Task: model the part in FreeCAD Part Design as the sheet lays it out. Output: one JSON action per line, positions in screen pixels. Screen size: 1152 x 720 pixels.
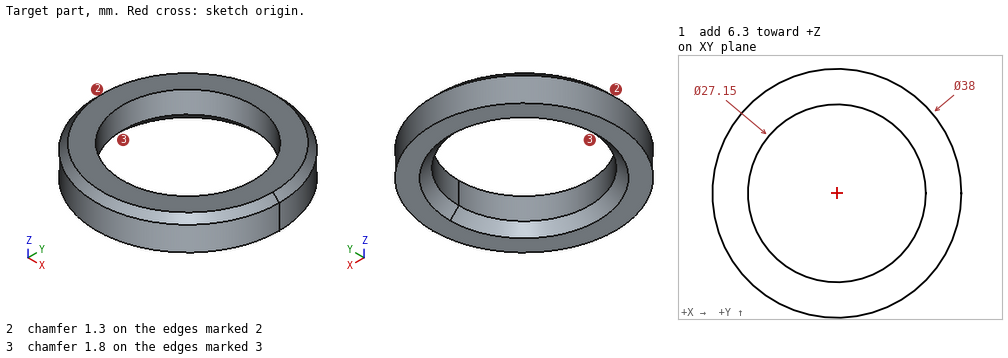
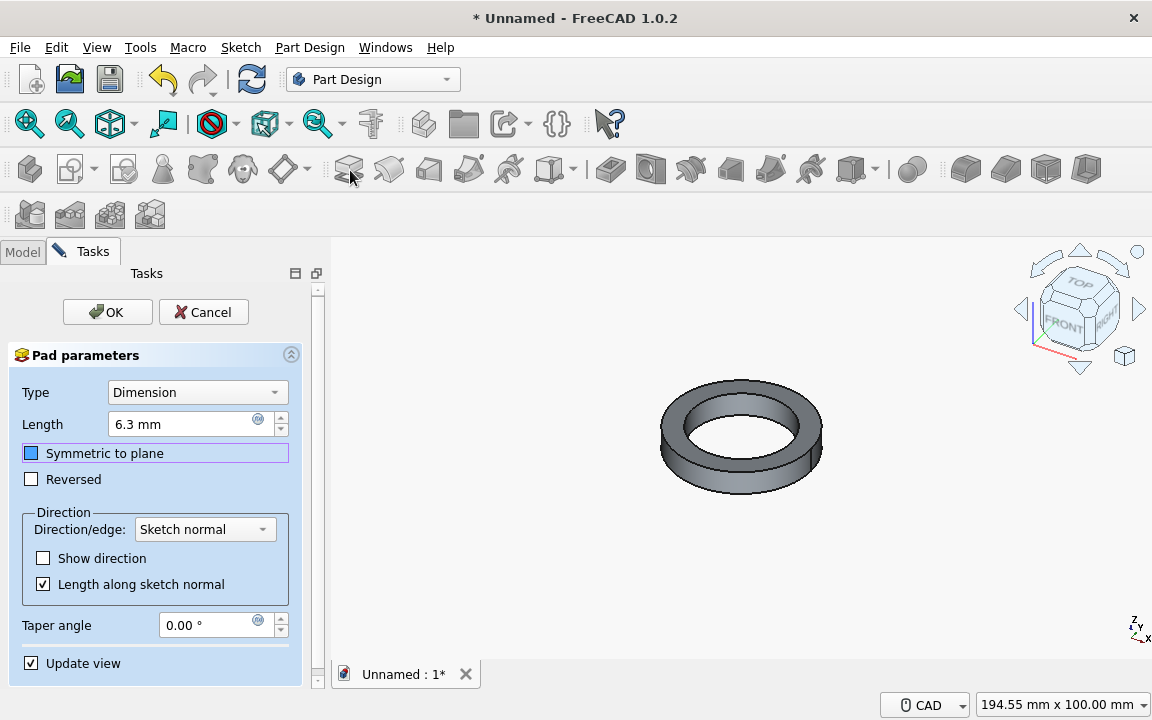
{"action": "left_click", "coordinate": [108, 312]}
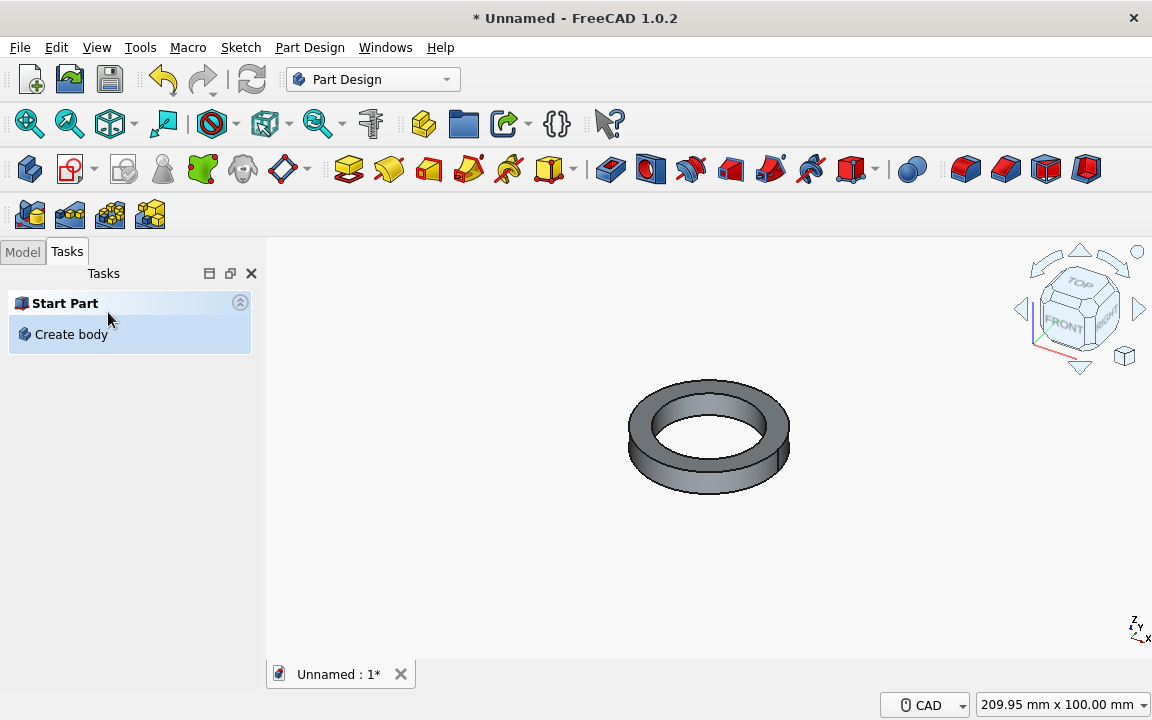
{"action": "key", "text": "v f"}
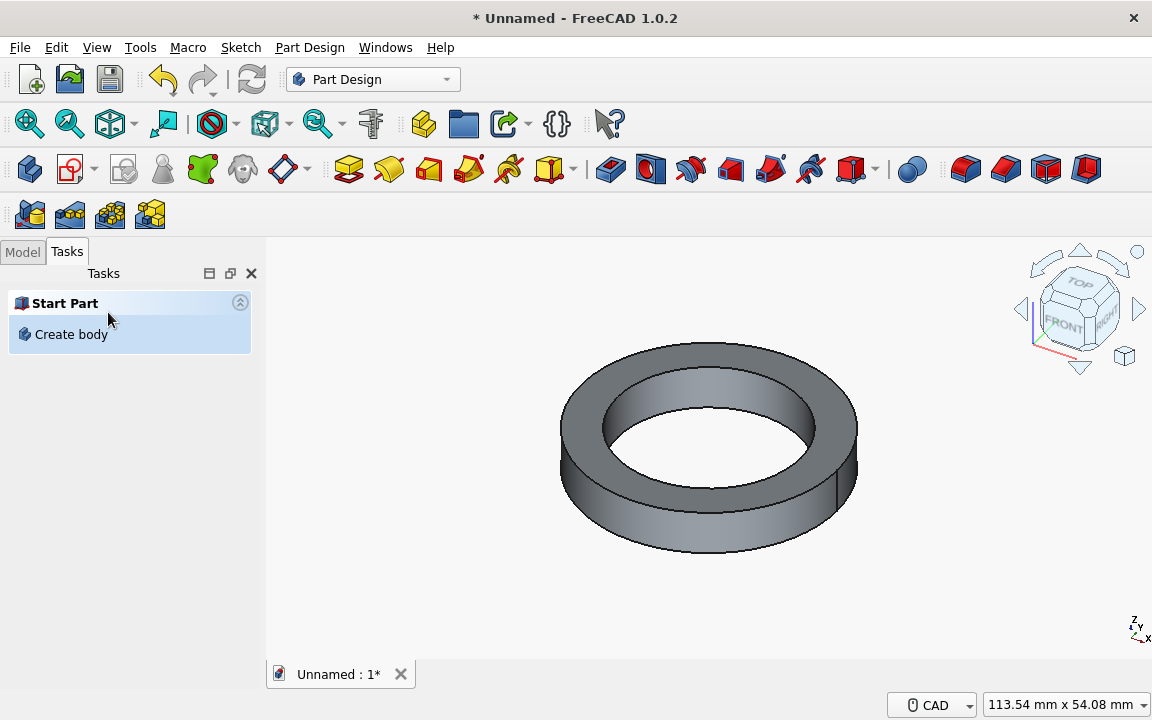
{"action": "left_click", "coordinate": [561, 436]}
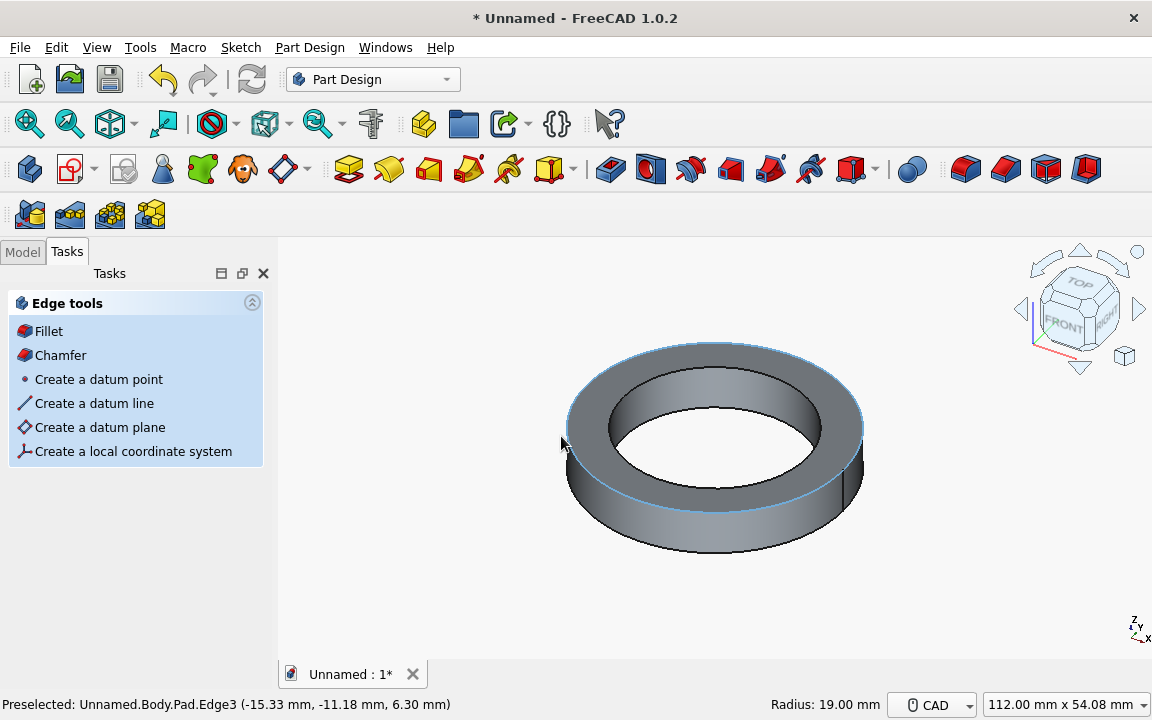
{"action": "left_click", "coordinate": [1006, 170]}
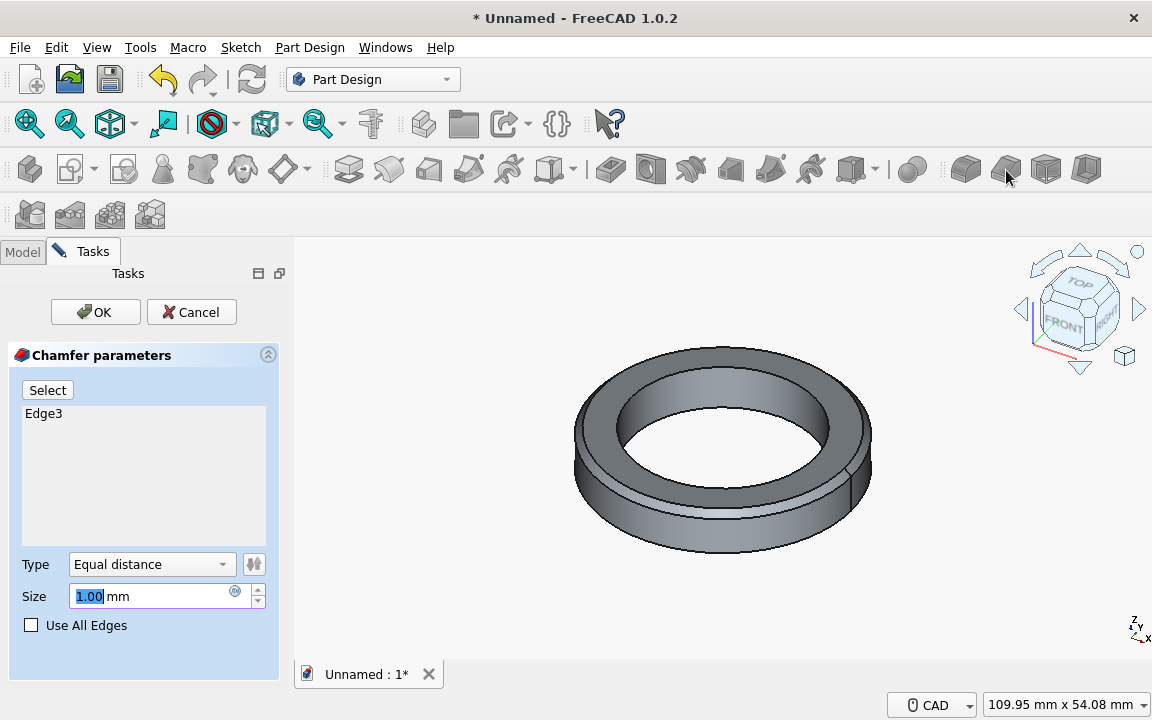
{"action": "type", "text": "1.3"}
{"action": "key", "text": "Tab"}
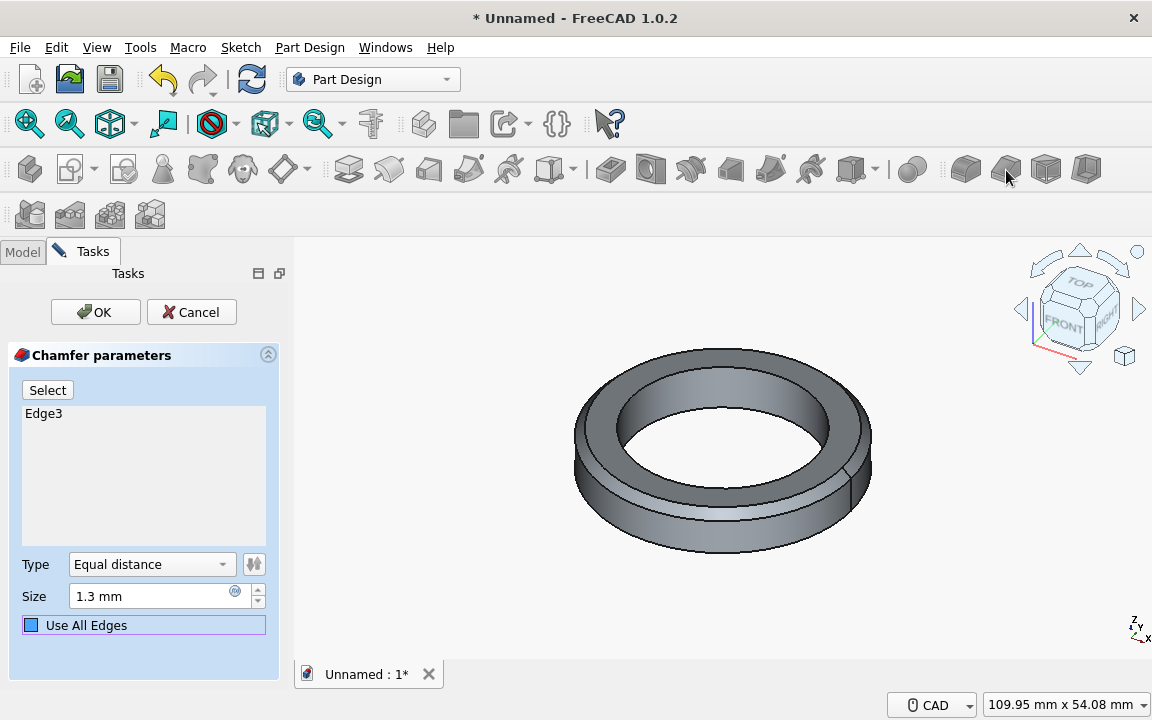
{"action": "left_click", "coordinate": [96, 312]}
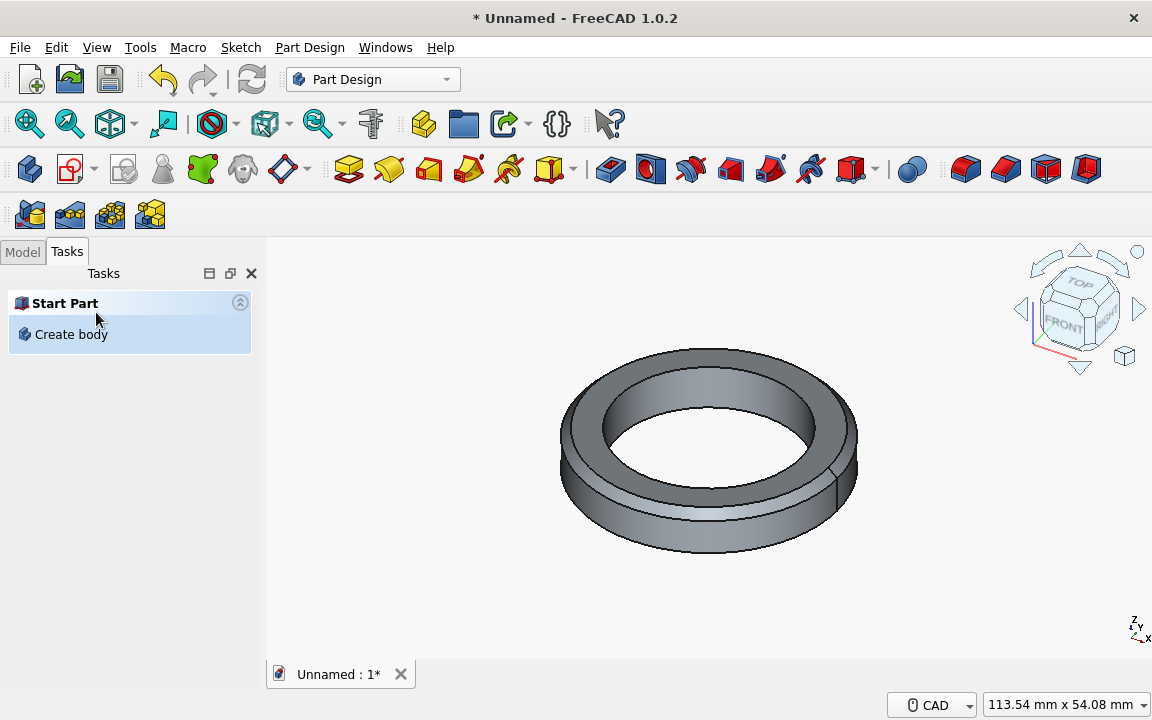
{"action": "key", "text": "0"}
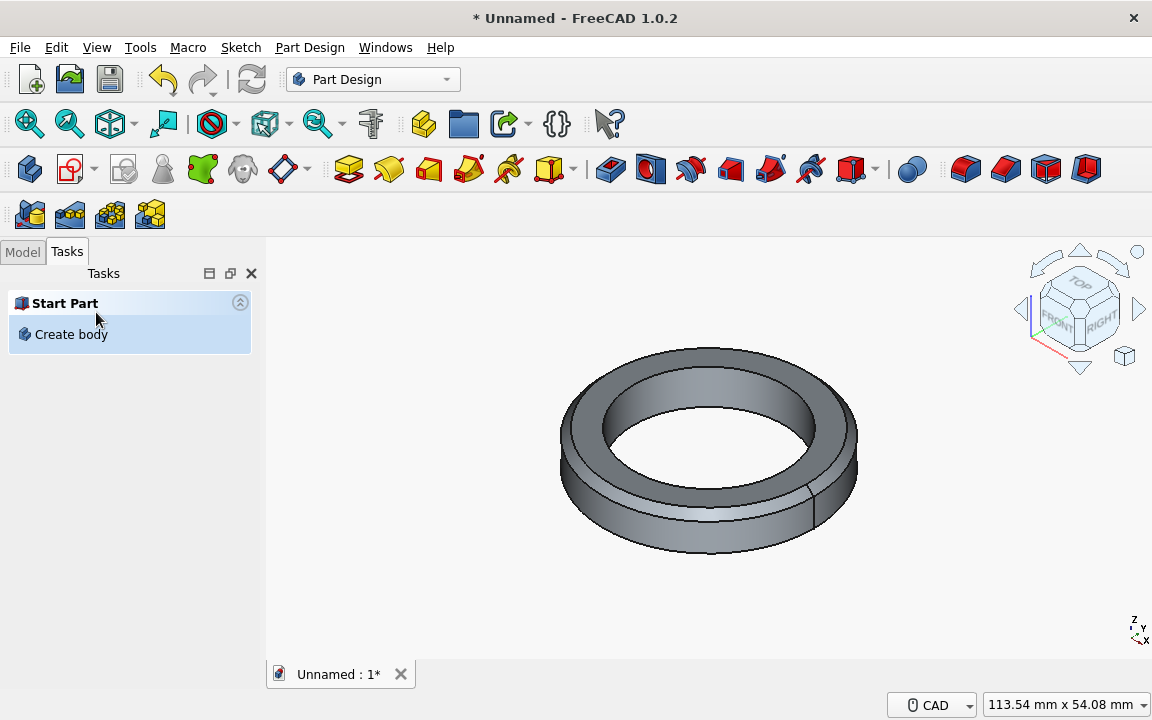
{"action": "key", "text": "2"}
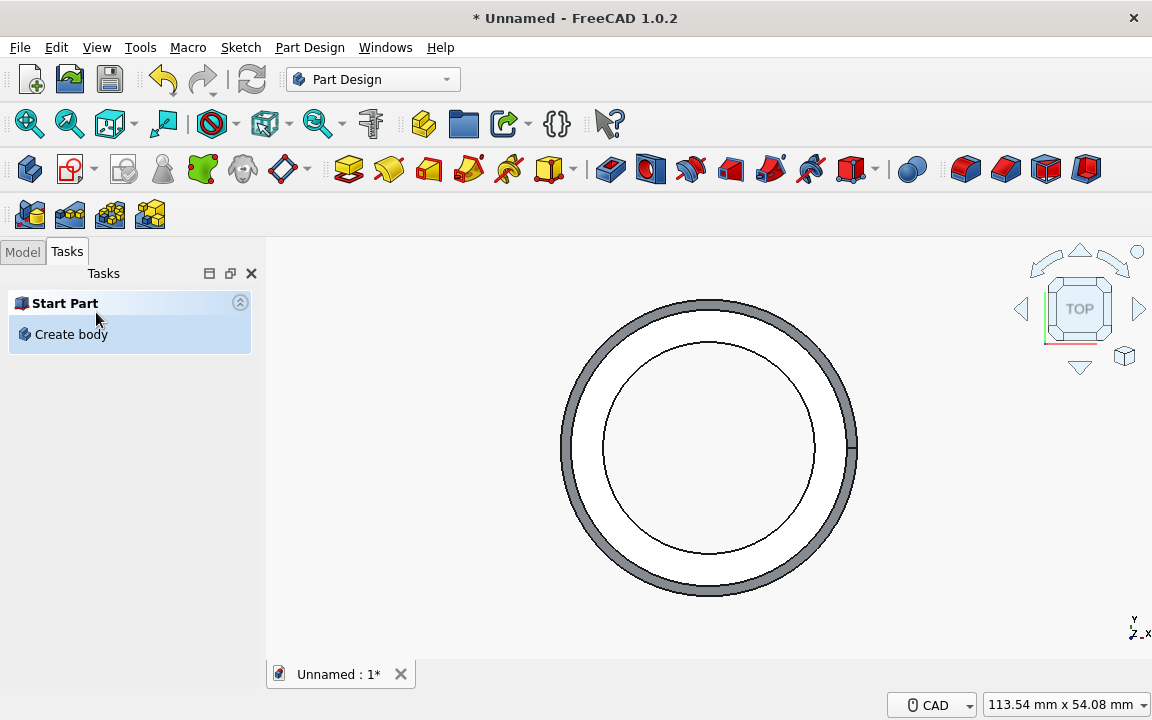
{"action": "key", "text": "1"}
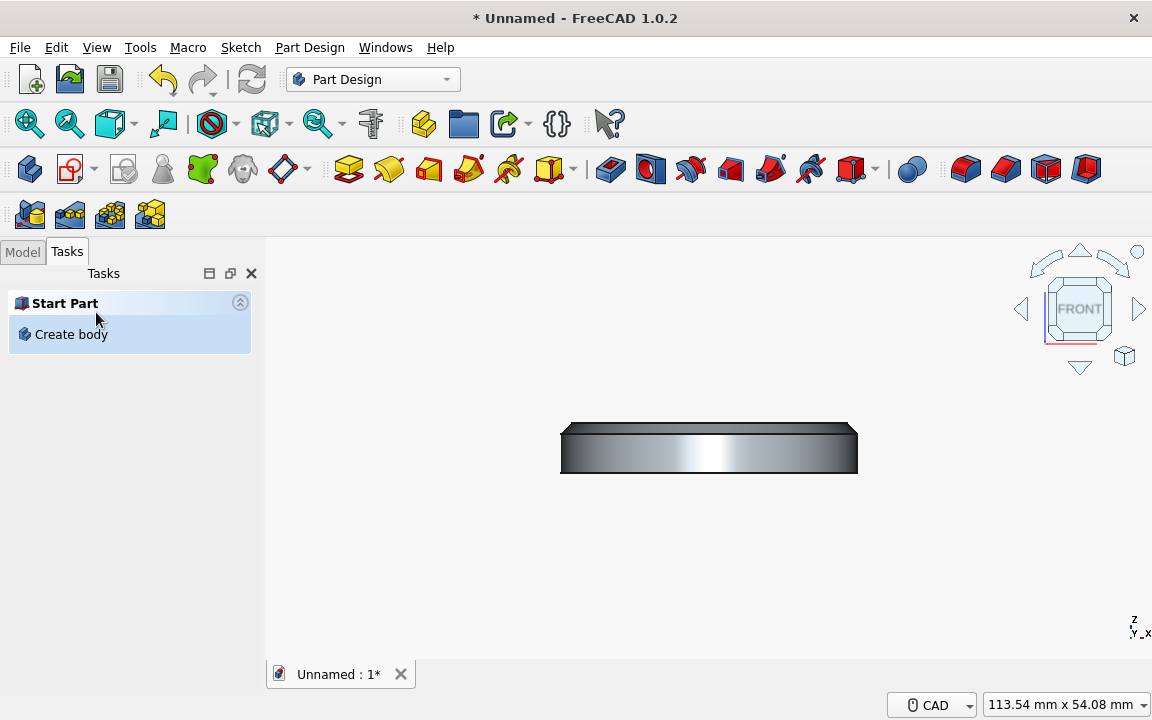
{"action": "key", "text": "v f"}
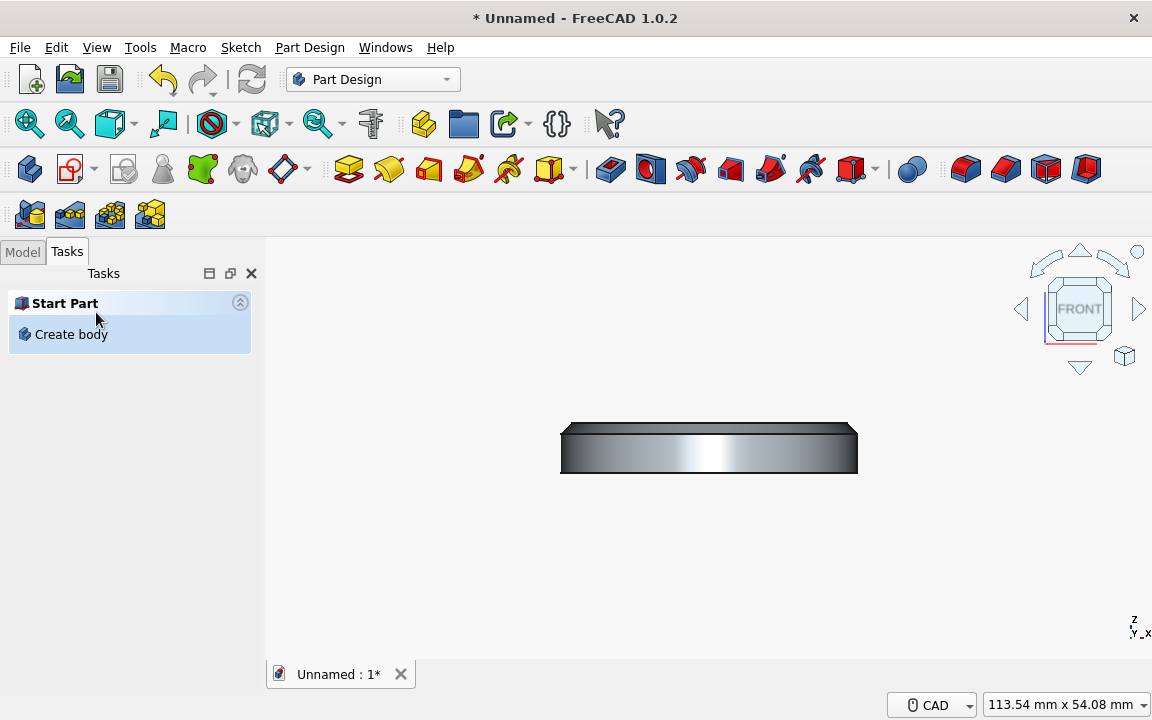
{"action": "key", "text": "3"}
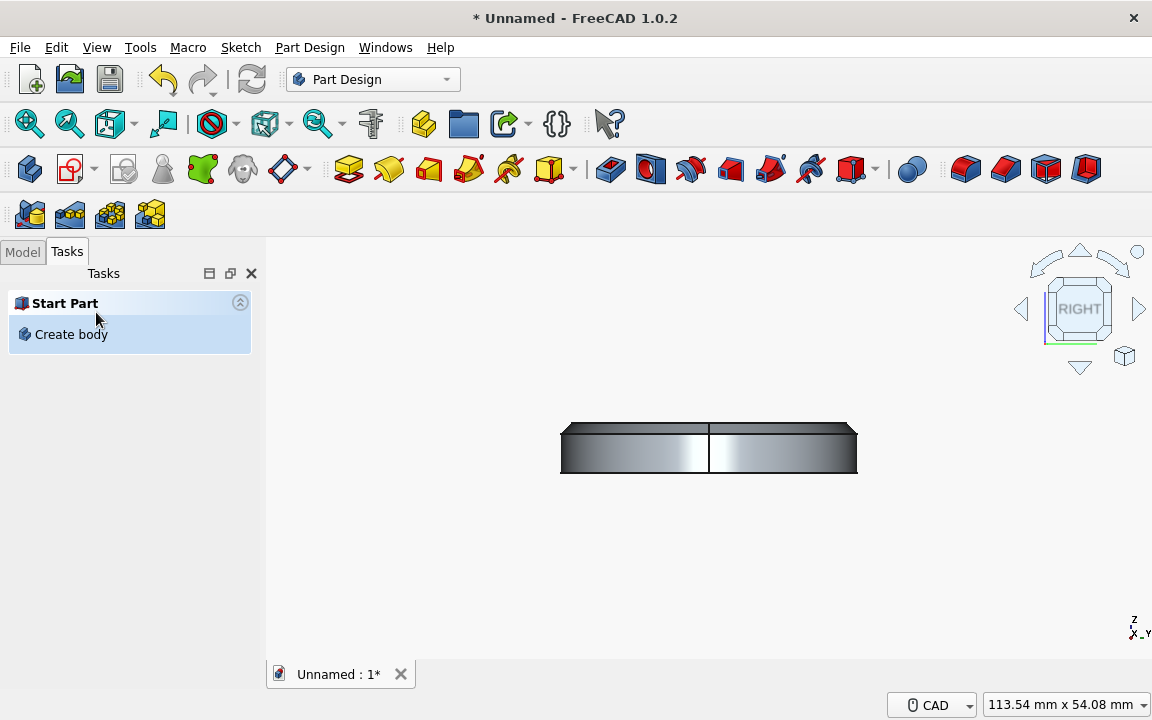
{"action": "key", "text": "v f"}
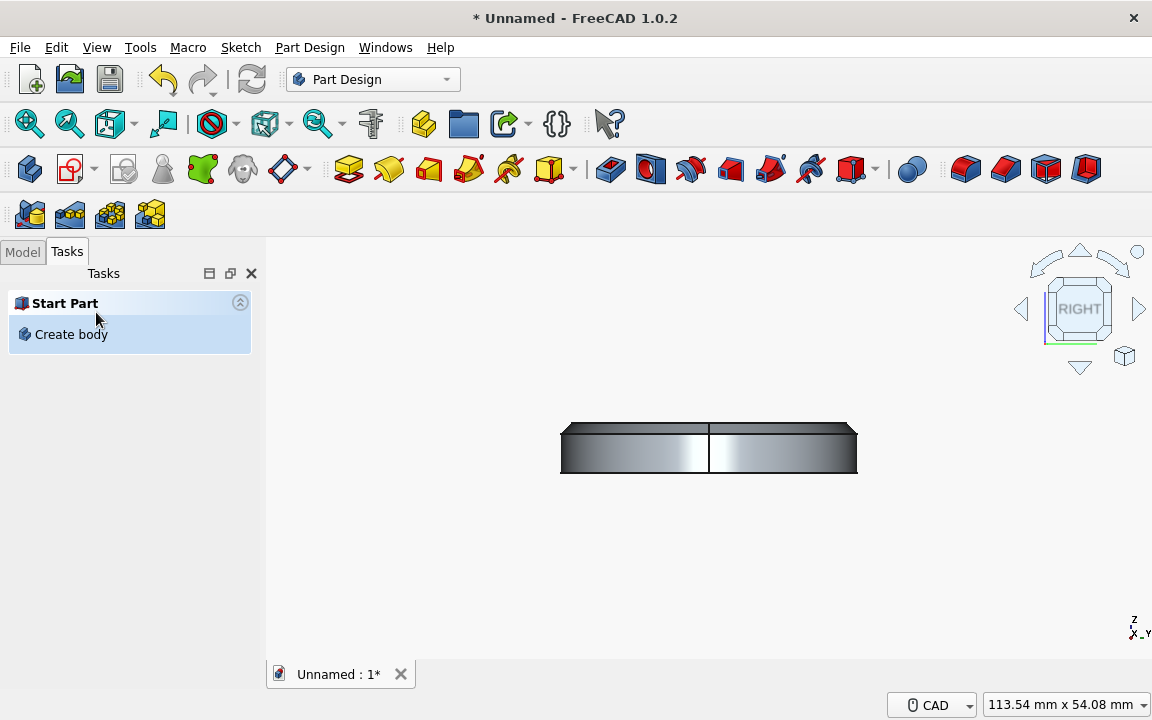
{"action": "key", "text": "5"}